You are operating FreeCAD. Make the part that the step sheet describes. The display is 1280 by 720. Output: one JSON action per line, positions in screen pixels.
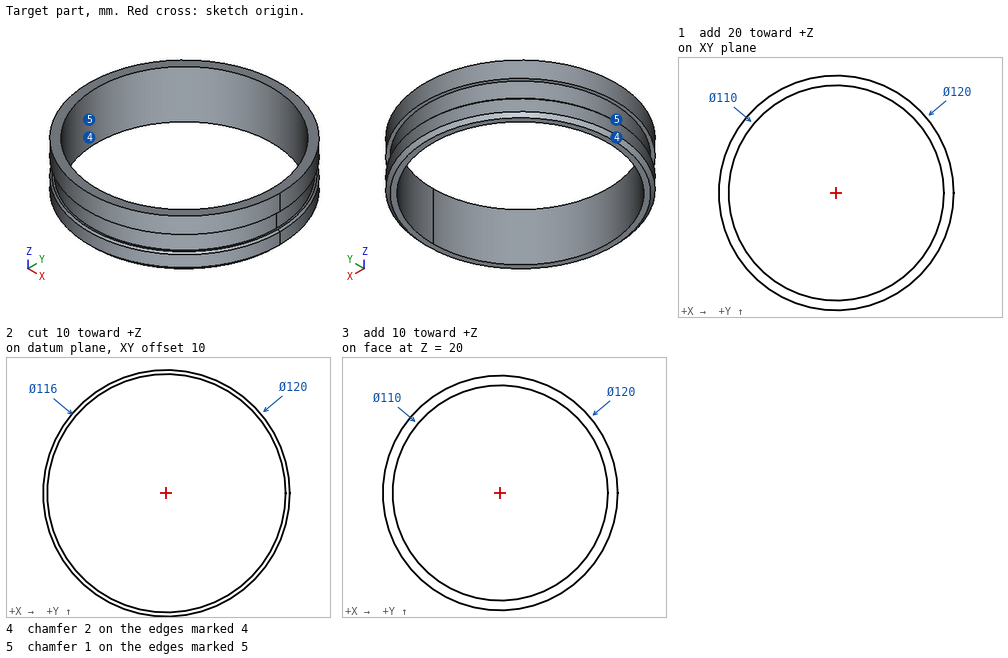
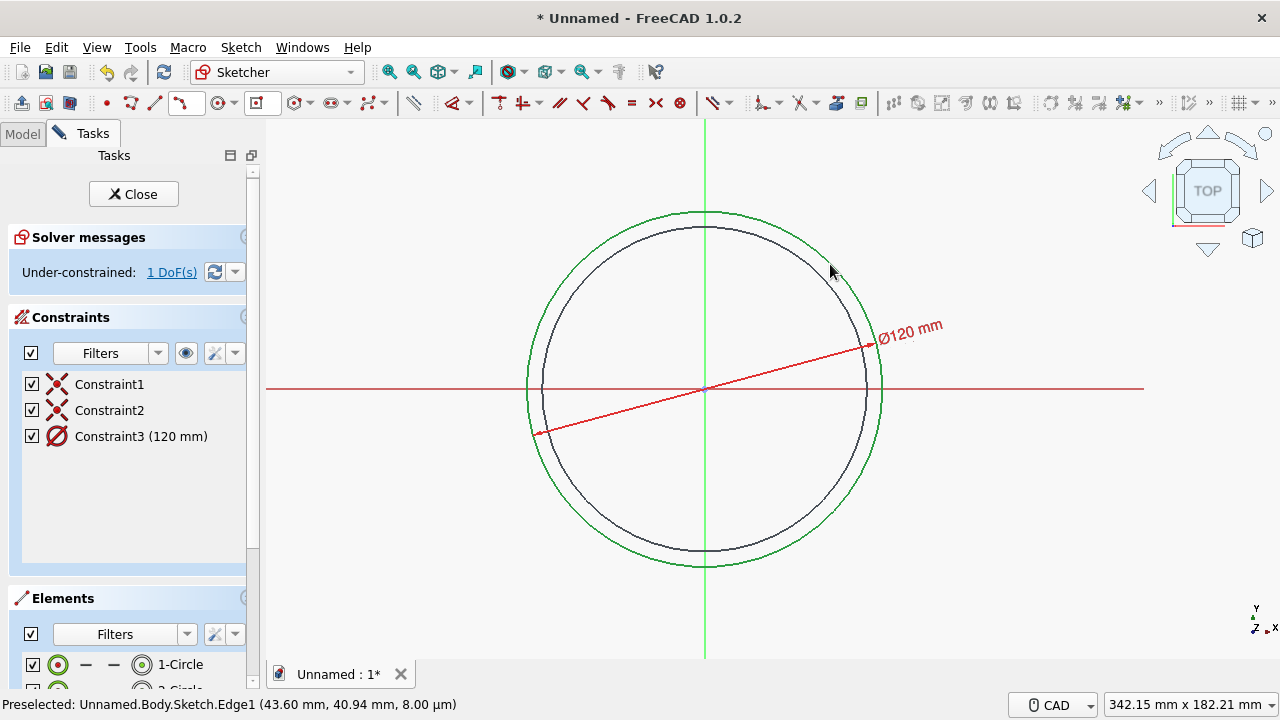
{"action": "left_click", "coordinate": [819, 274]}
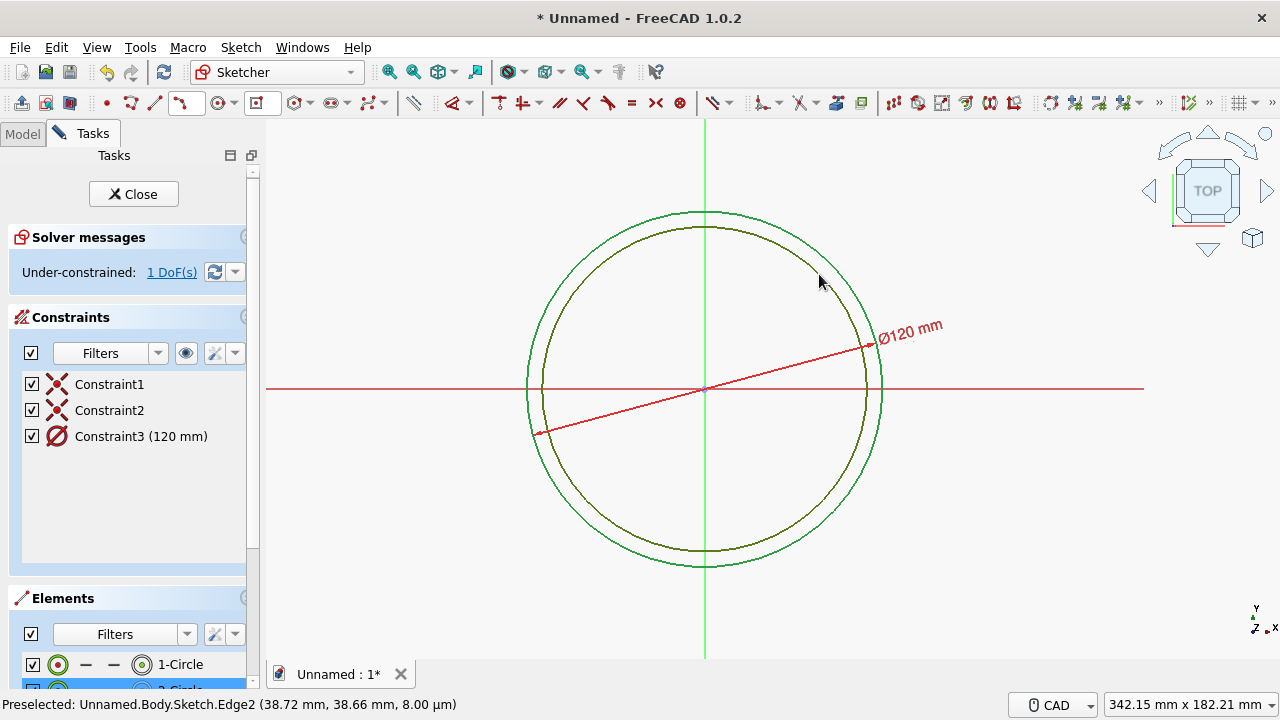
{"action": "key", "text": "k o"}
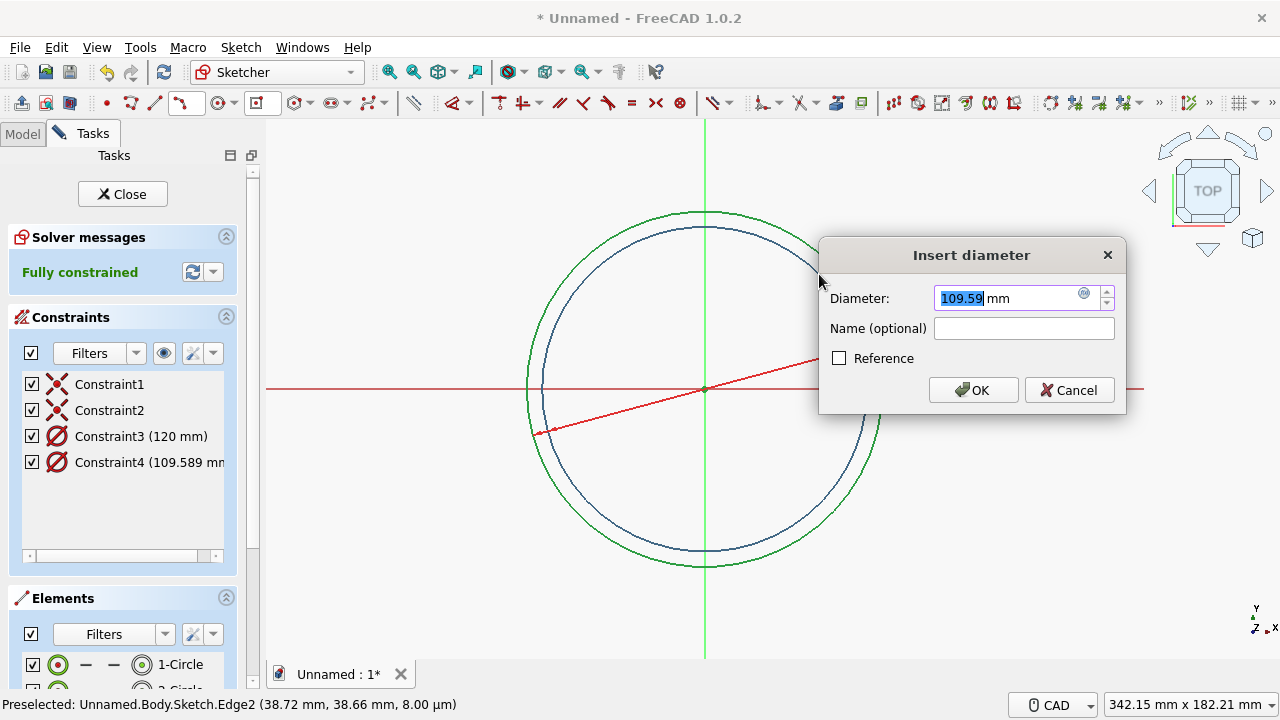
{"action": "type", "text": "110"}
{"action": "key", "text": "Return"}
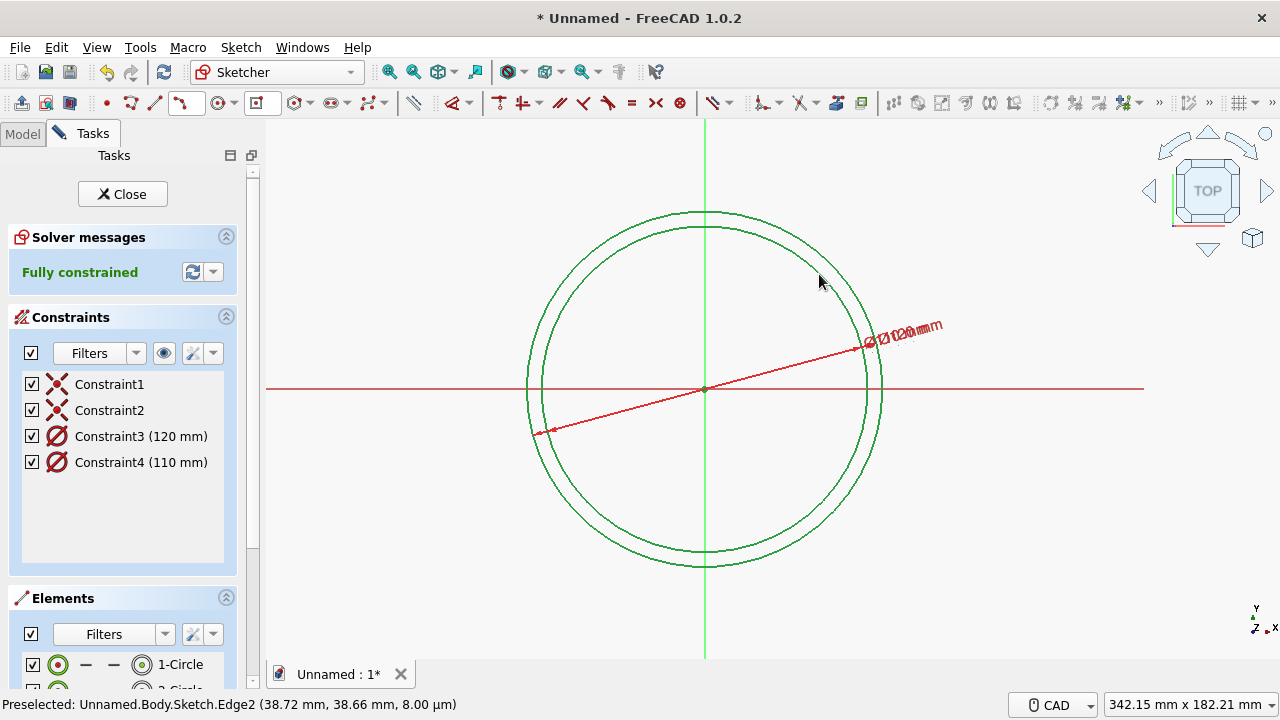
{"action": "left_click", "coordinate": [123, 194]}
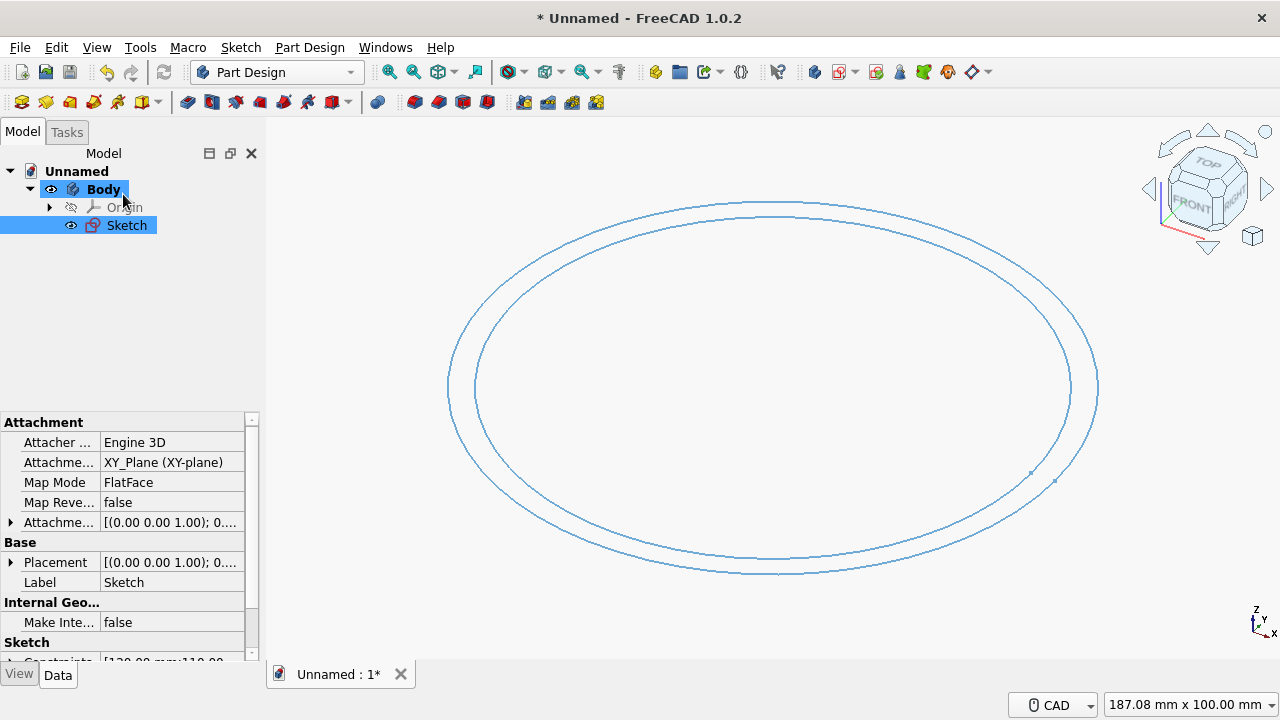
{"action": "left_click", "coordinate": [22, 102]}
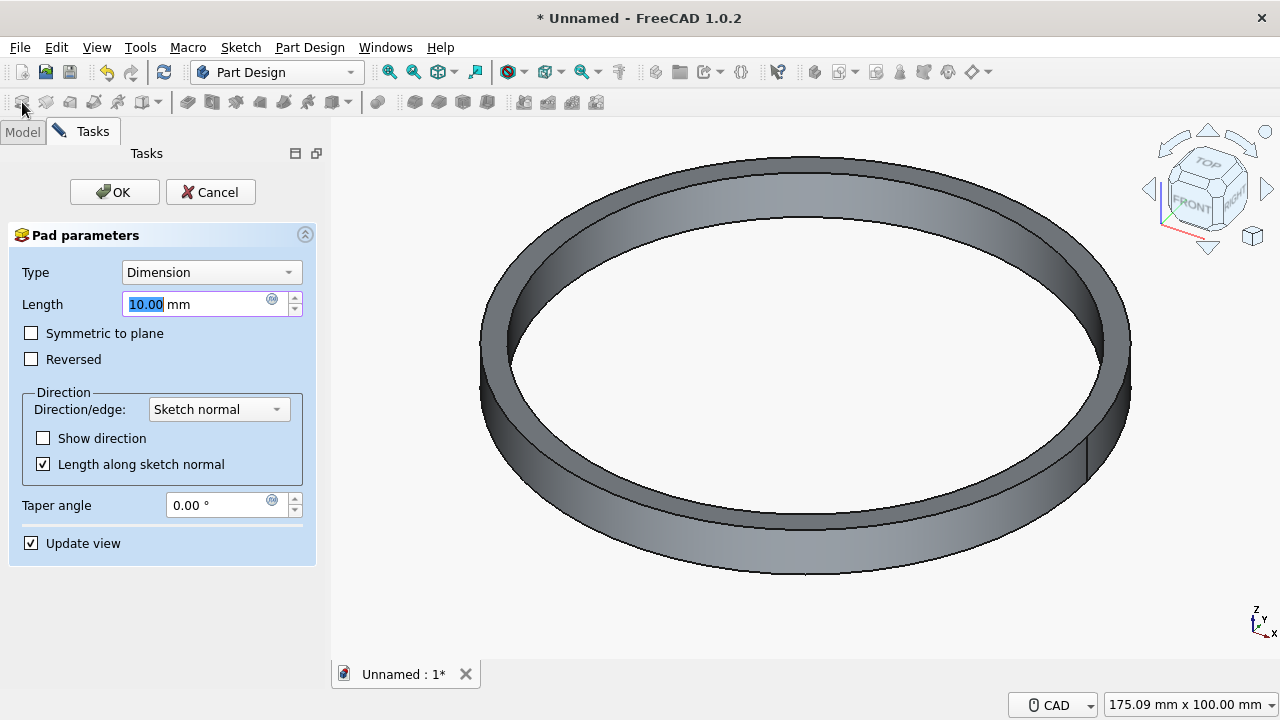
{"action": "type", "text": "20"}
{"action": "key", "text": "Tab"}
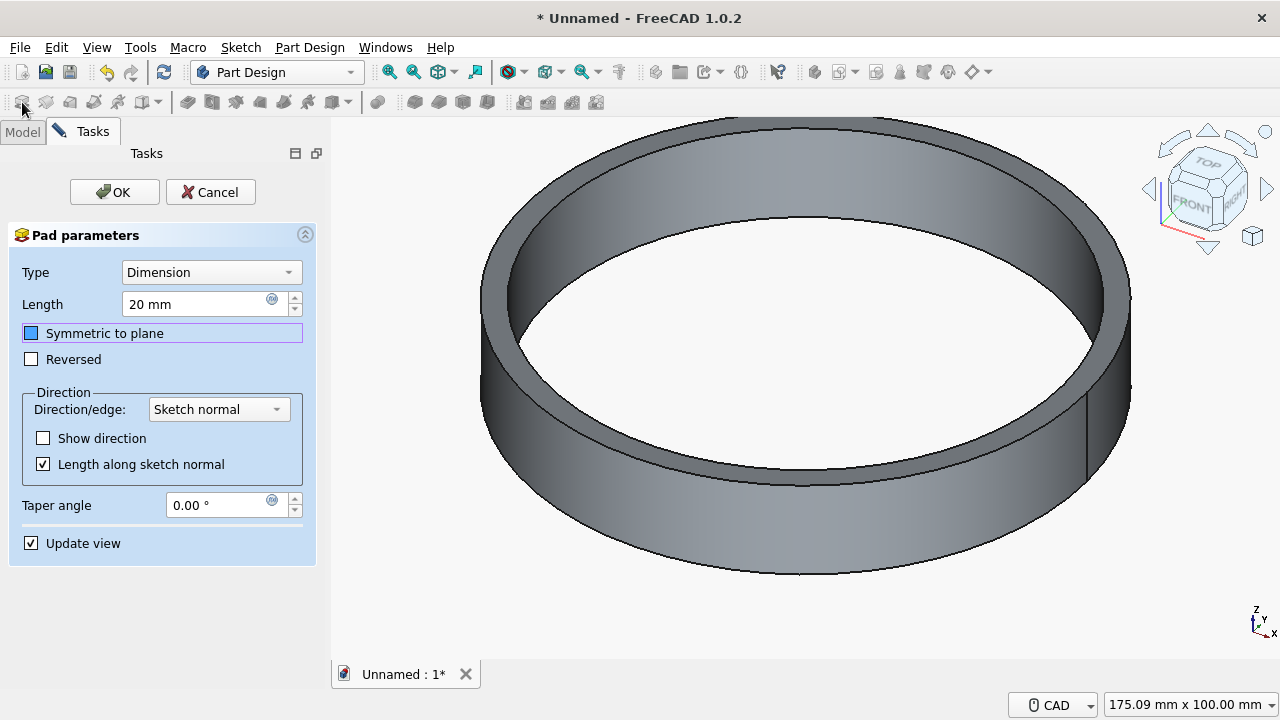
{"action": "left_click", "coordinate": [115, 192]}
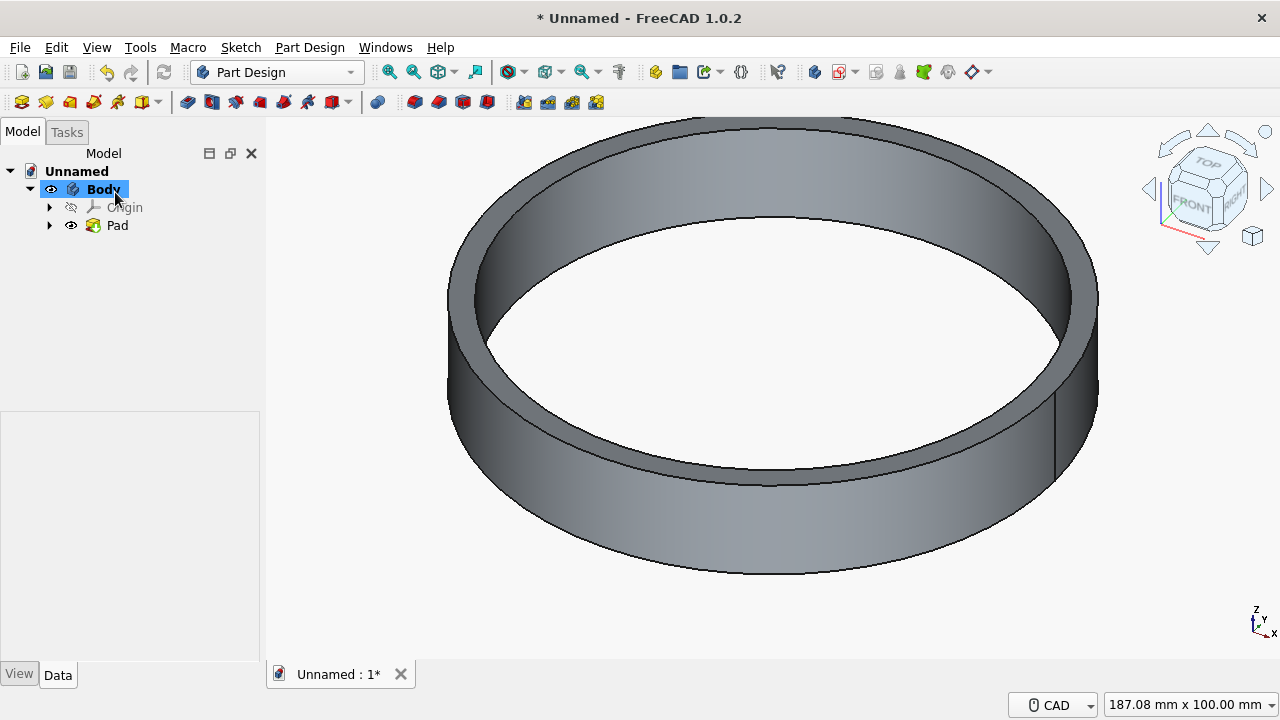
{"action": "left_click", "coordinate": [390, 72]}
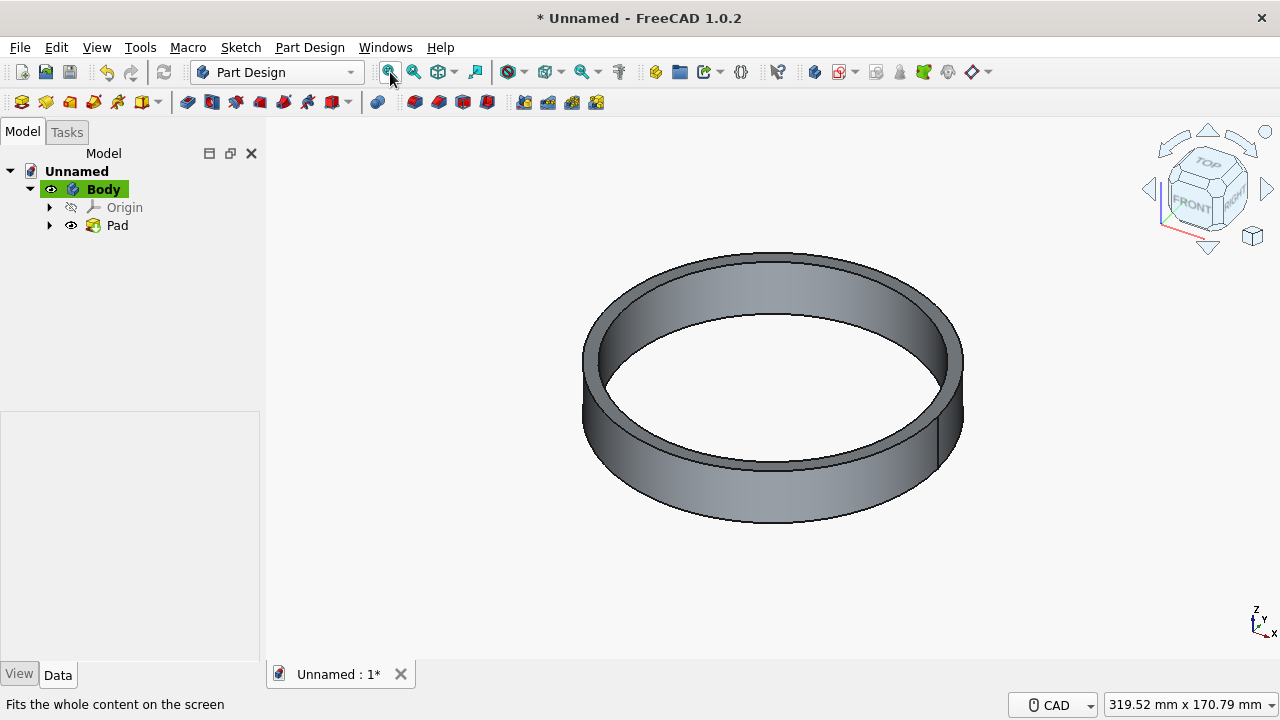
{"action": "left_click", "coordinate": [50, 207]}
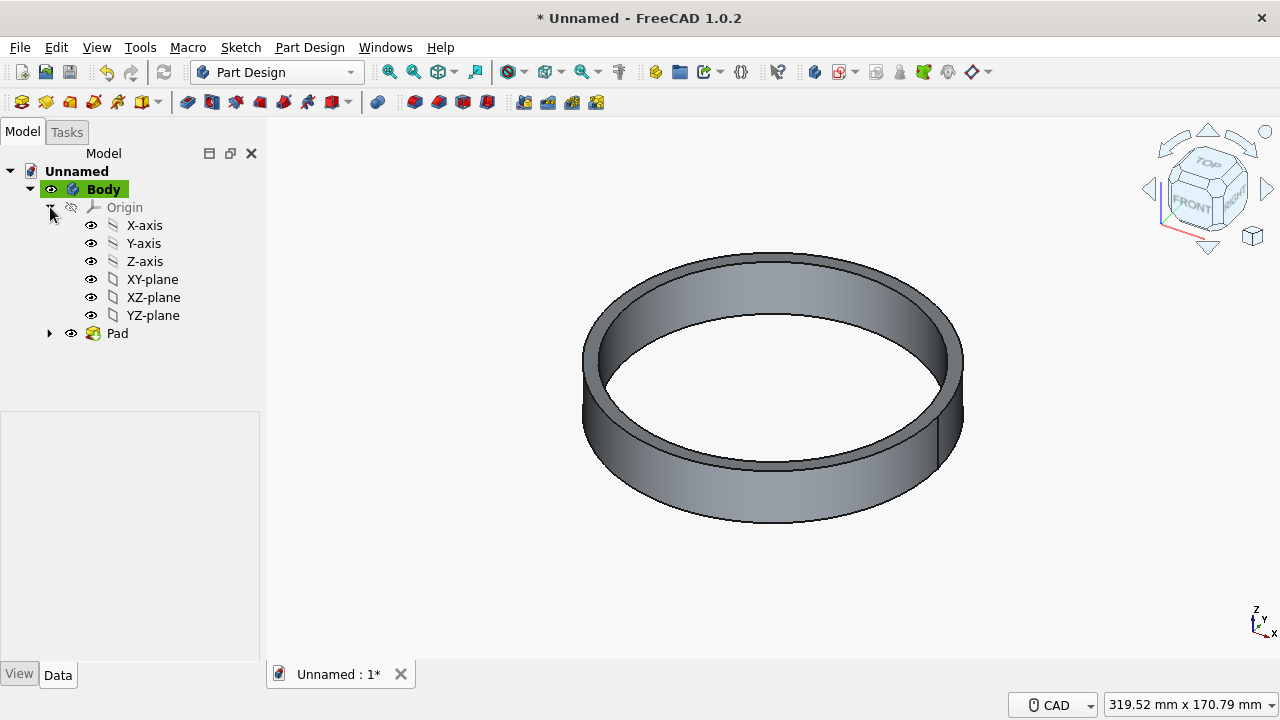
{"action": "left_click", "coordinate": [136, 279]}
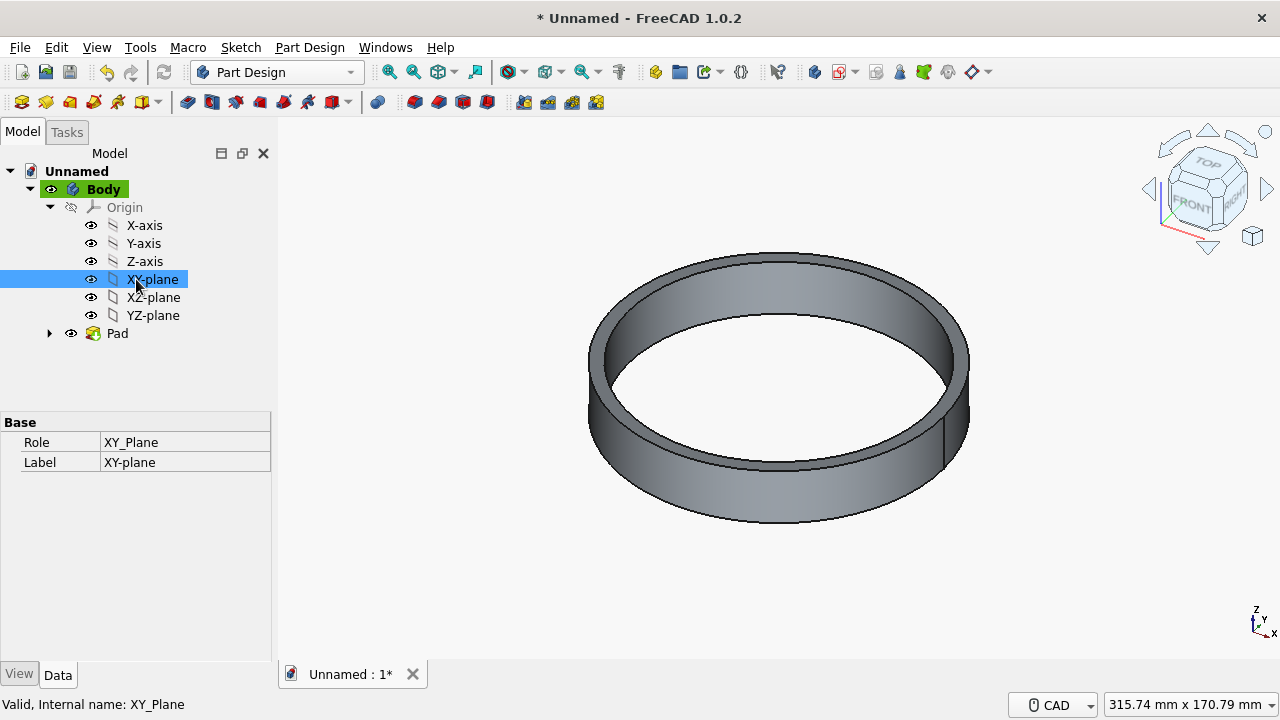
{"action": "left_click", "coordinate": [972, 72]}